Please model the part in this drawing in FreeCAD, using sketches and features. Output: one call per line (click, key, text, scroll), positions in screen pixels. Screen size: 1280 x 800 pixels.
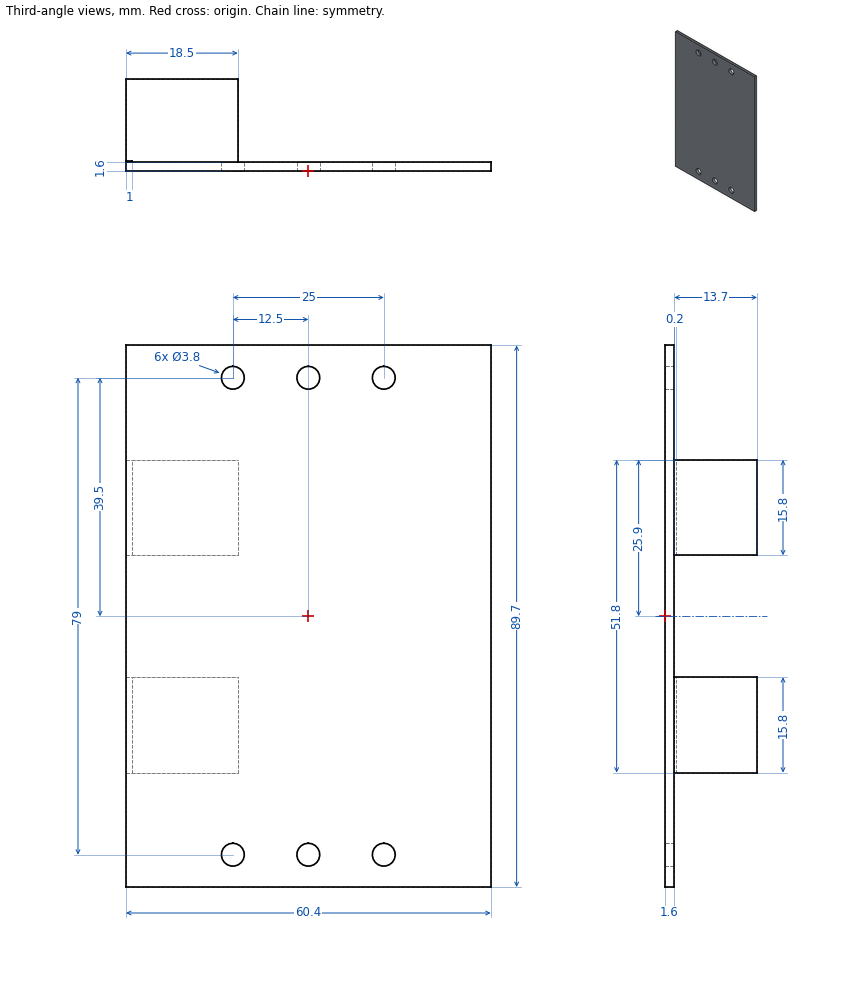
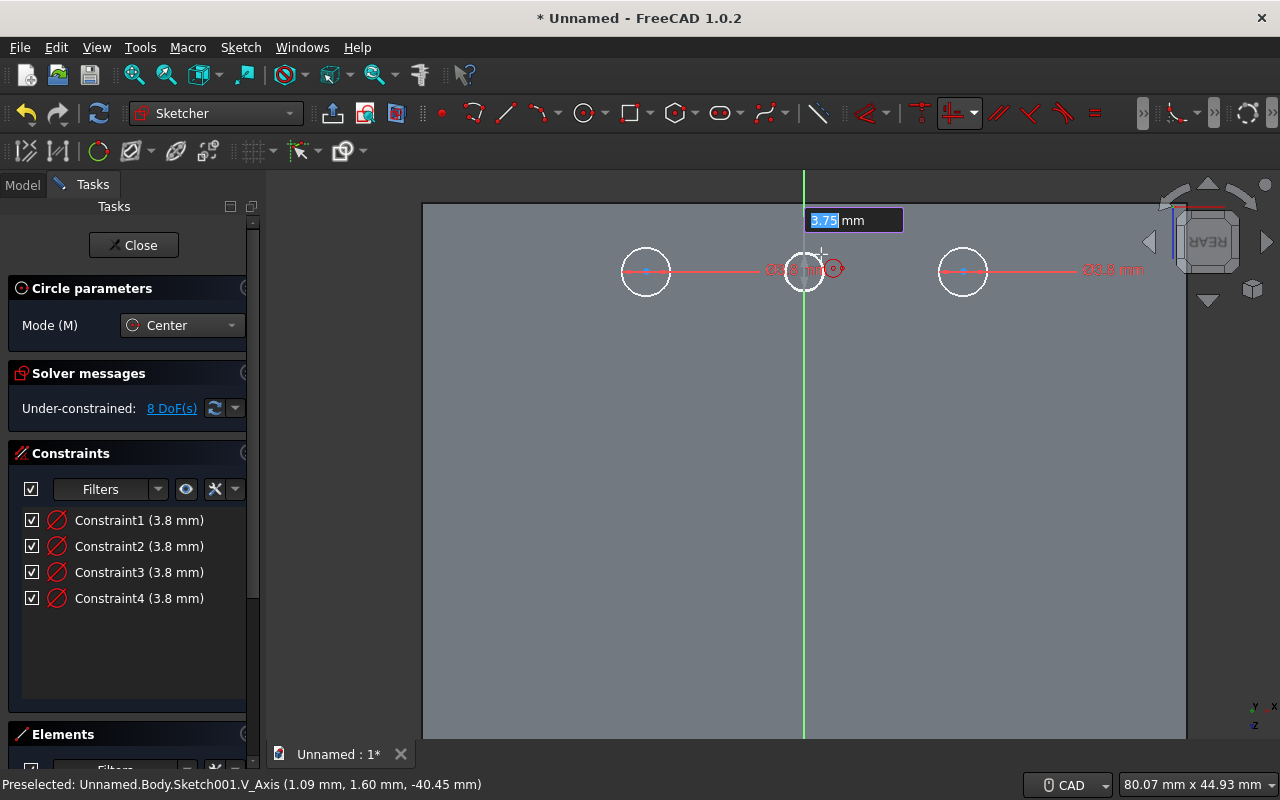
text(3.8)
key(Return)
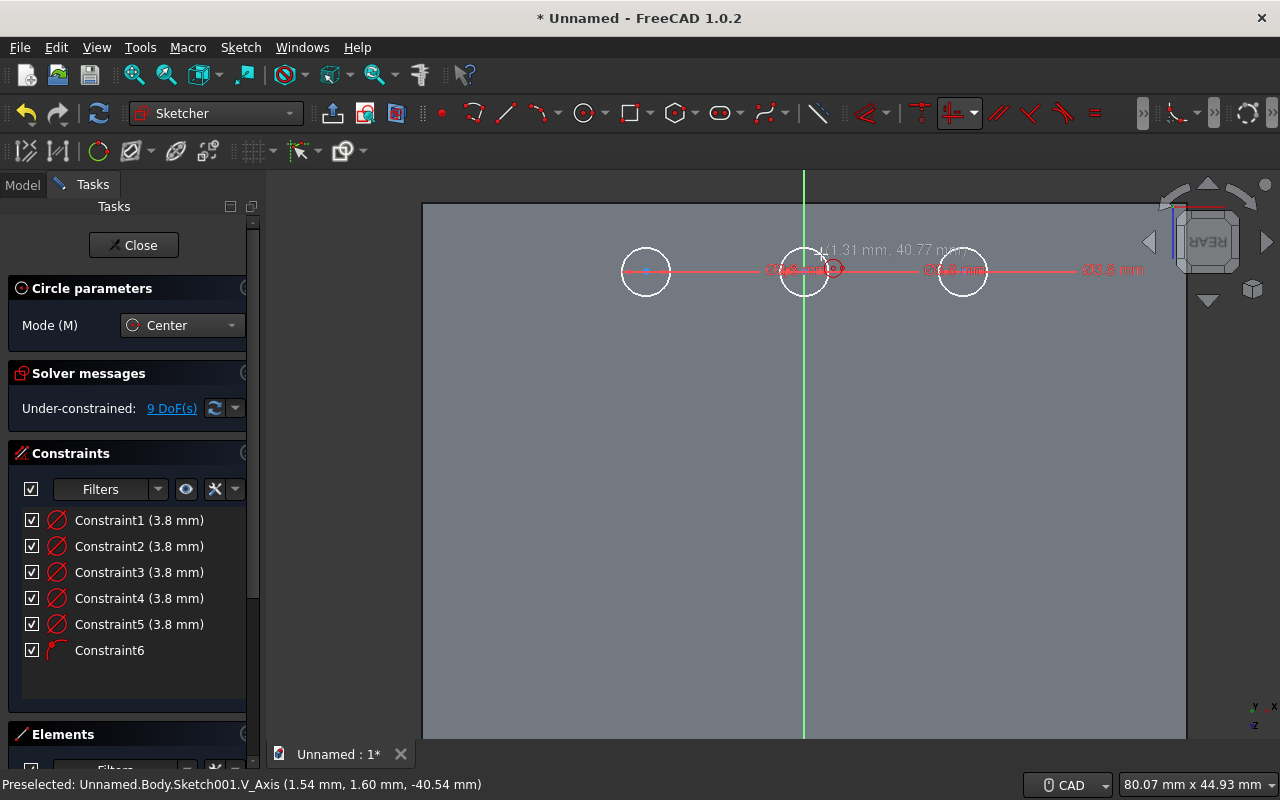
scroll(646, 270, down, 5)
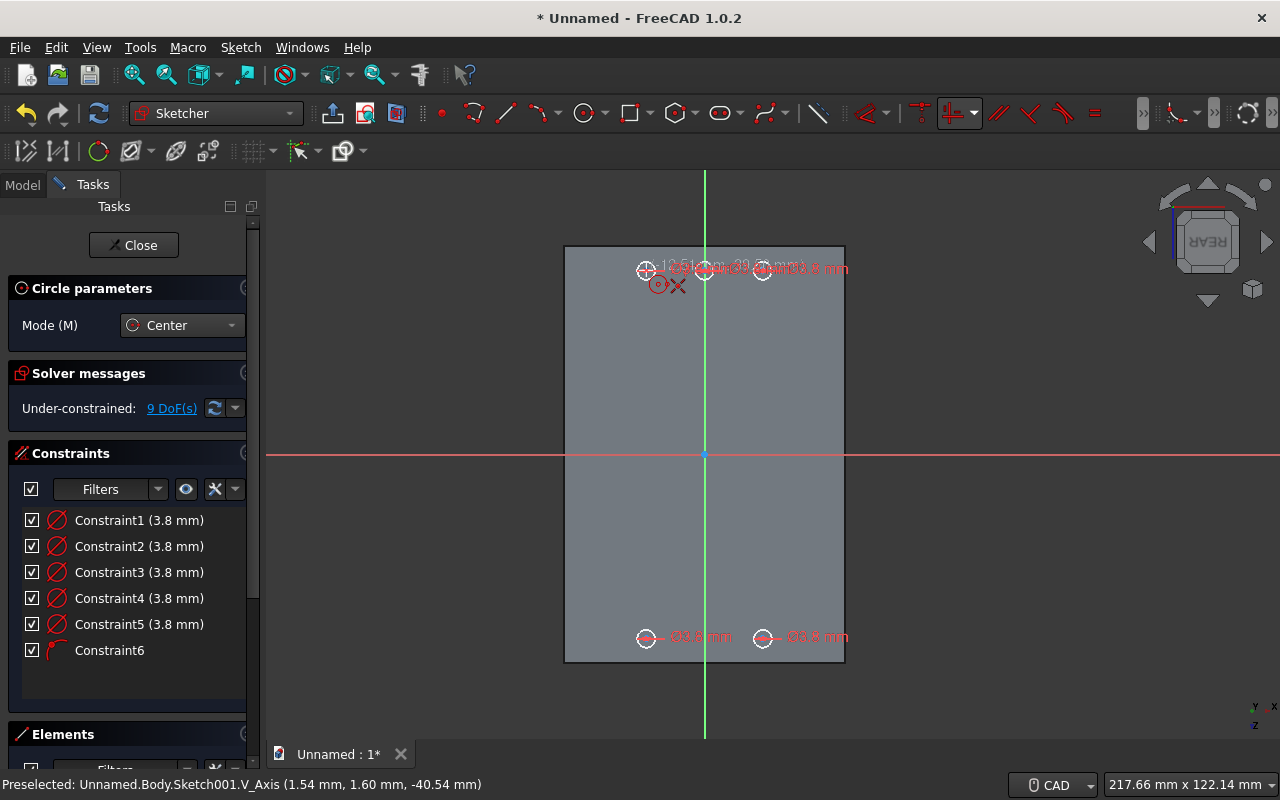
scroll(705, 639, up, 5)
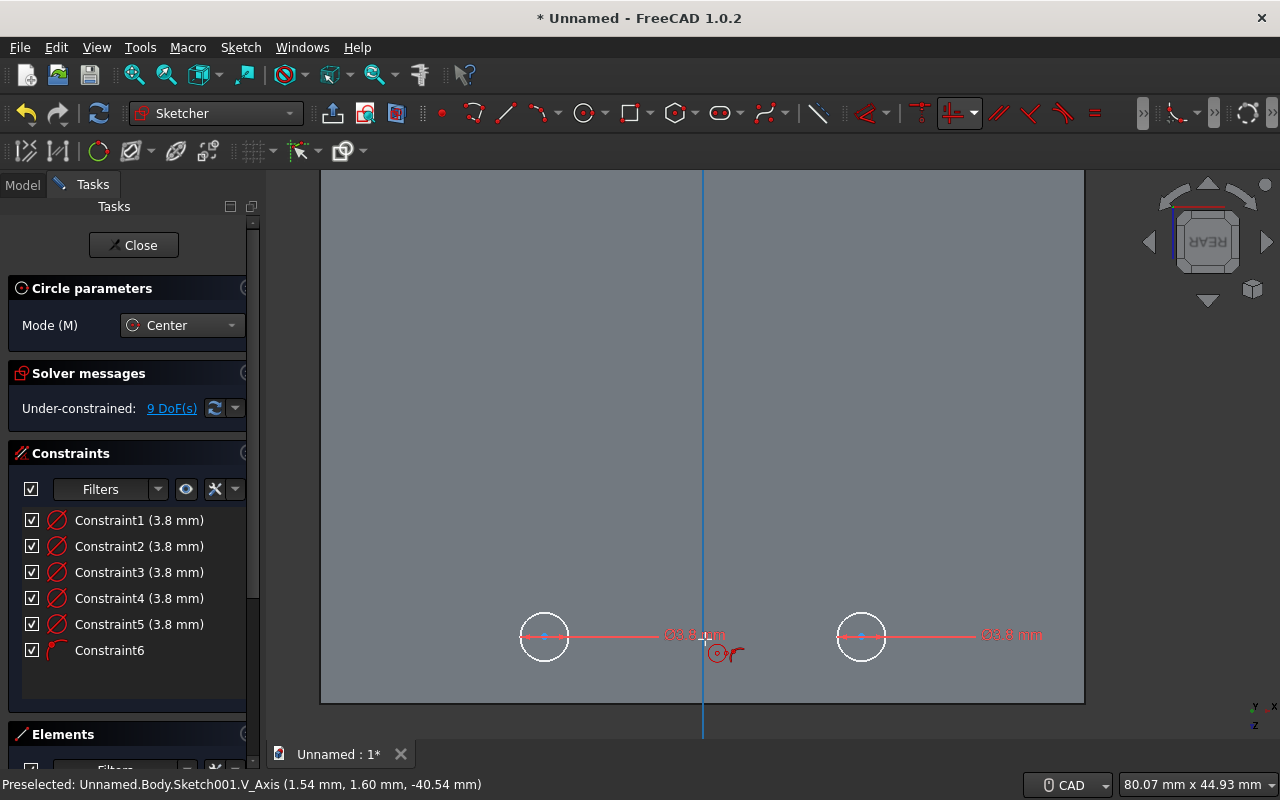
click(703, 636)
move(720, 619)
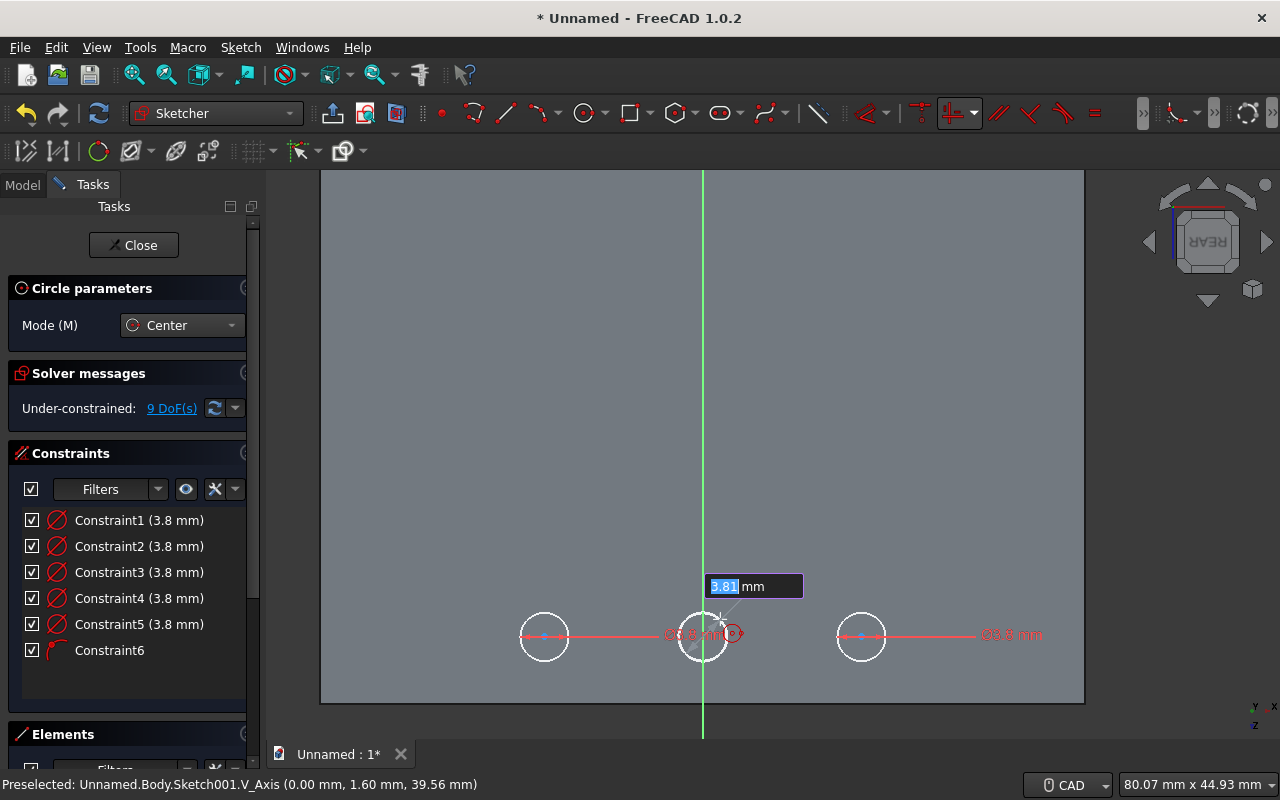
text(3.8)
key(Return)
key(Escape)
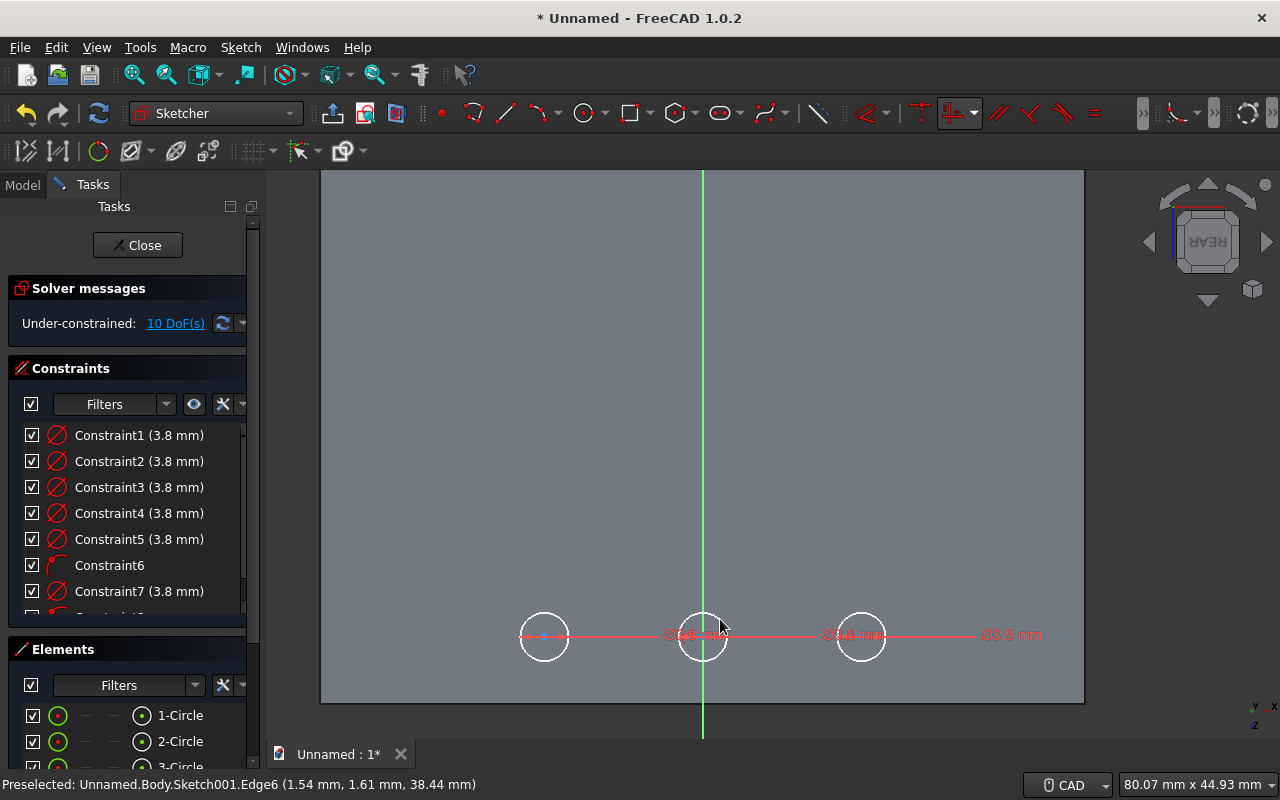
click(545, 637)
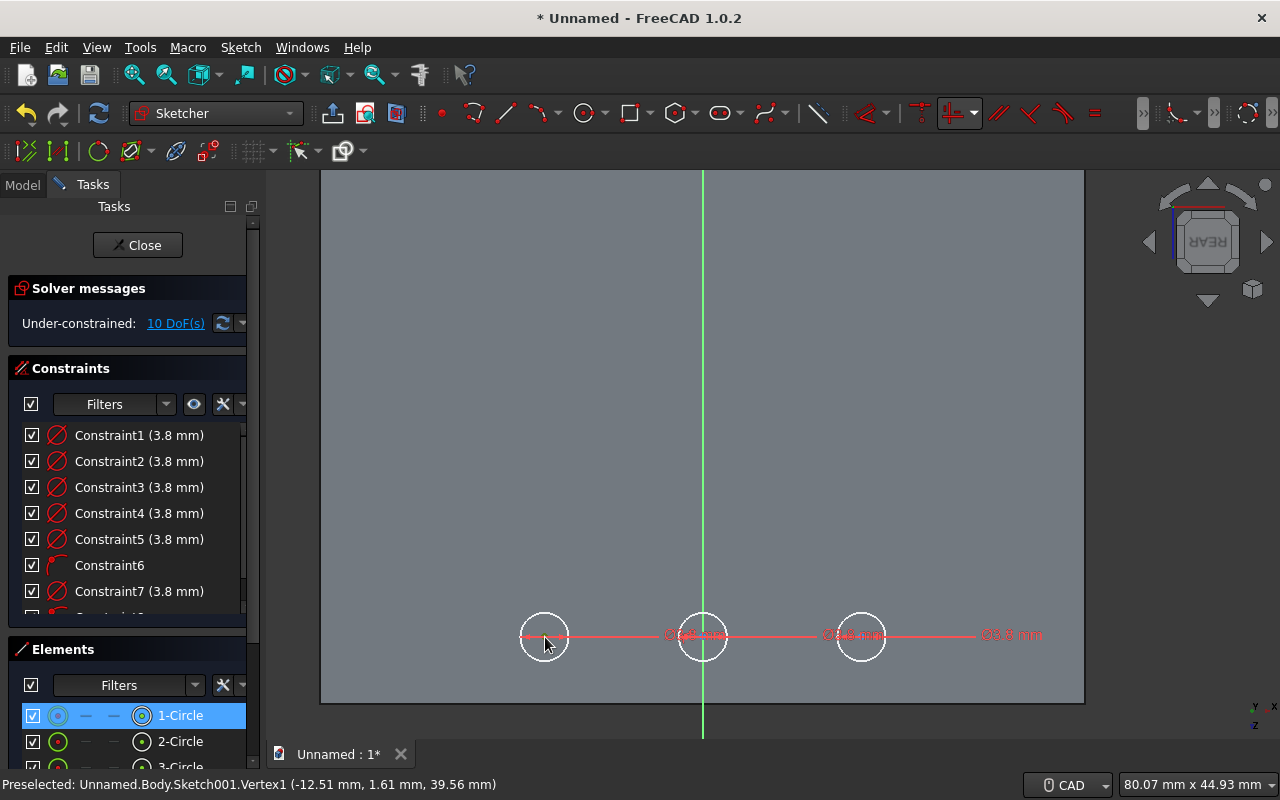
click(862, 637)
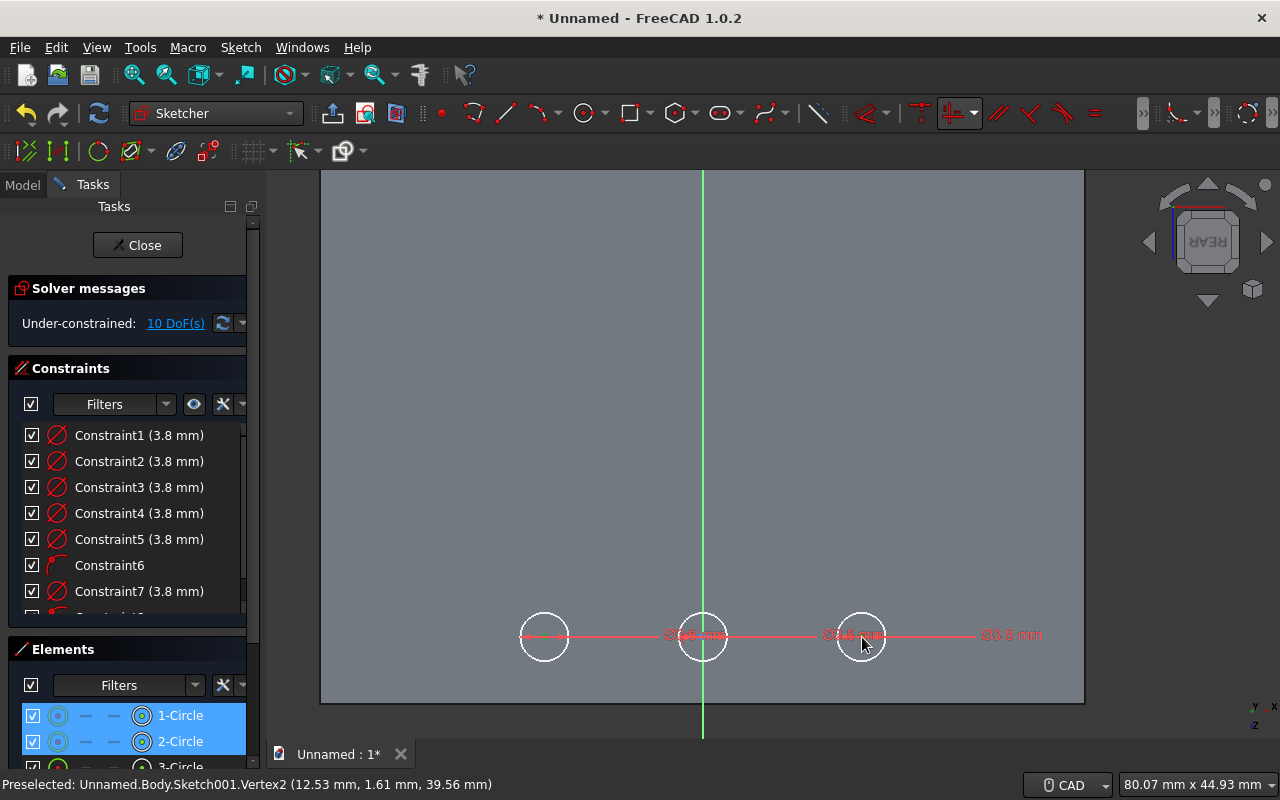
key(h)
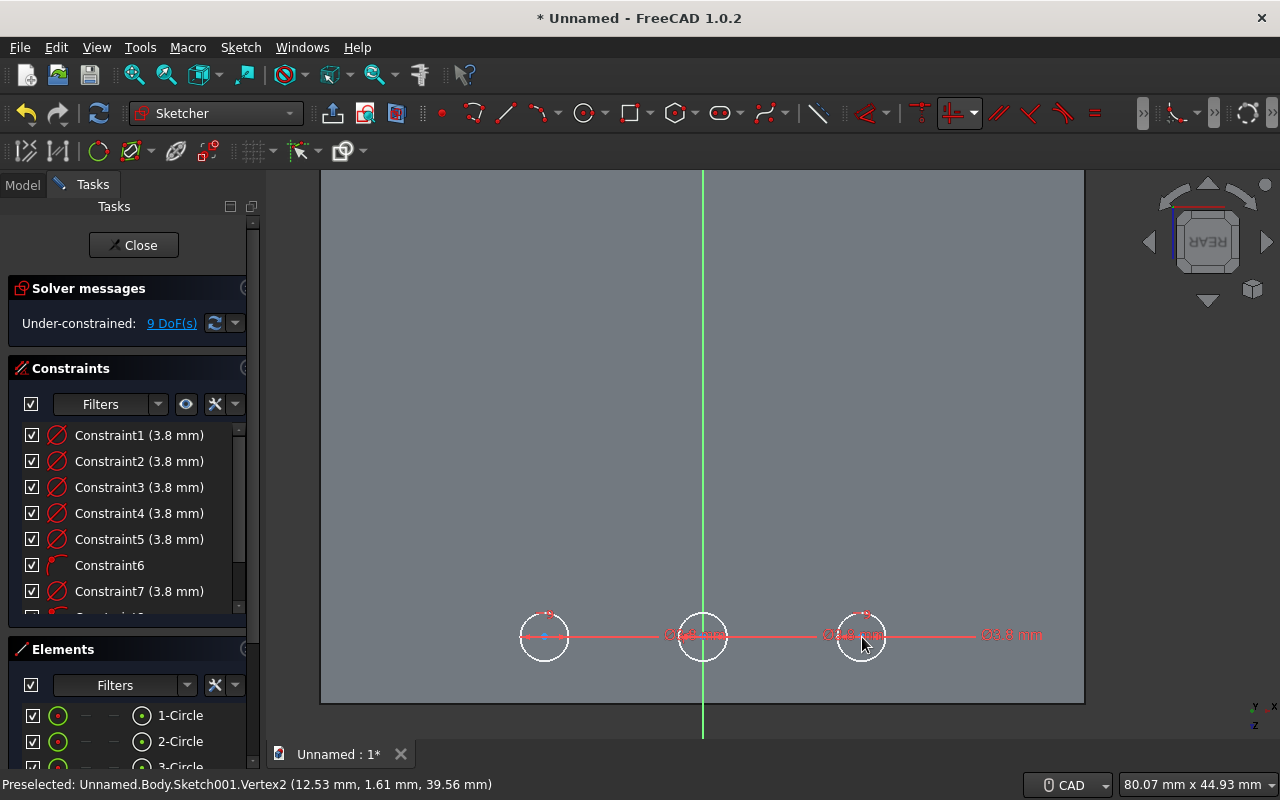
click(545, 637)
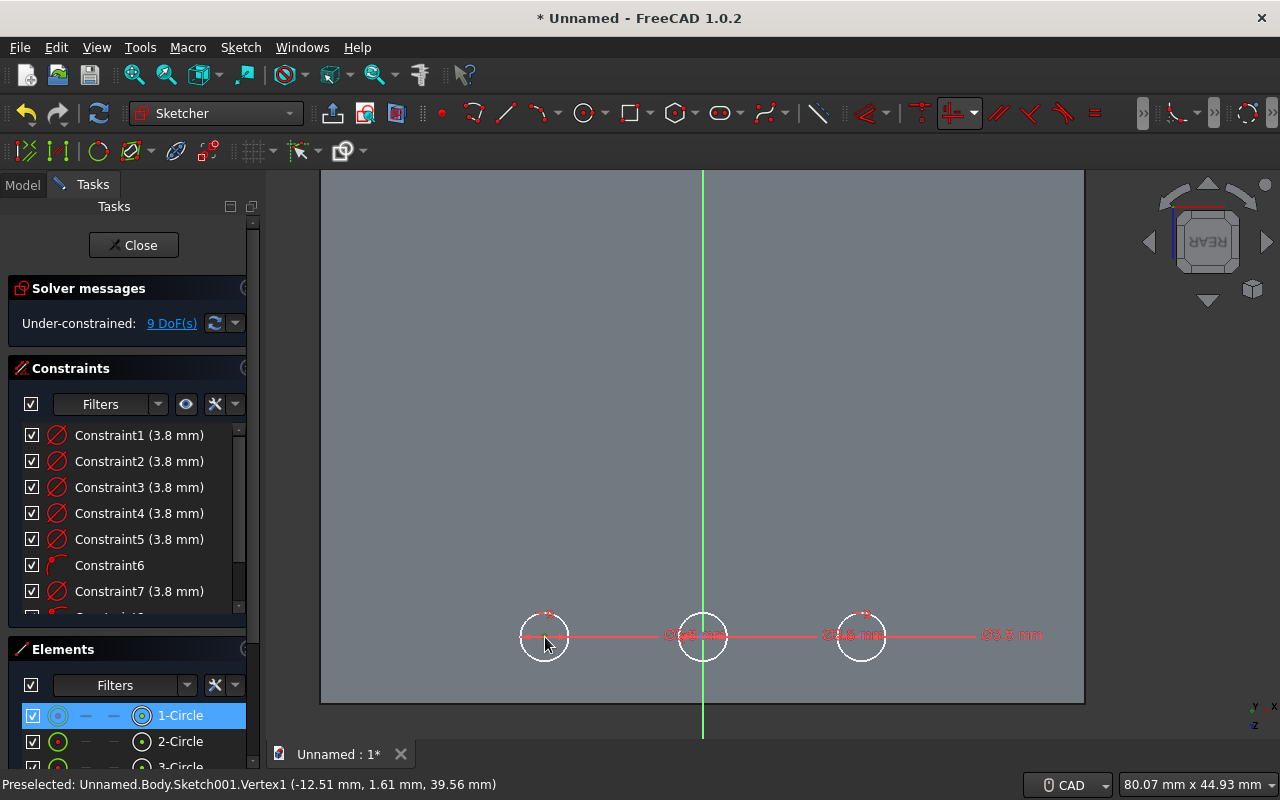
scroll(705, 640, down, 5)